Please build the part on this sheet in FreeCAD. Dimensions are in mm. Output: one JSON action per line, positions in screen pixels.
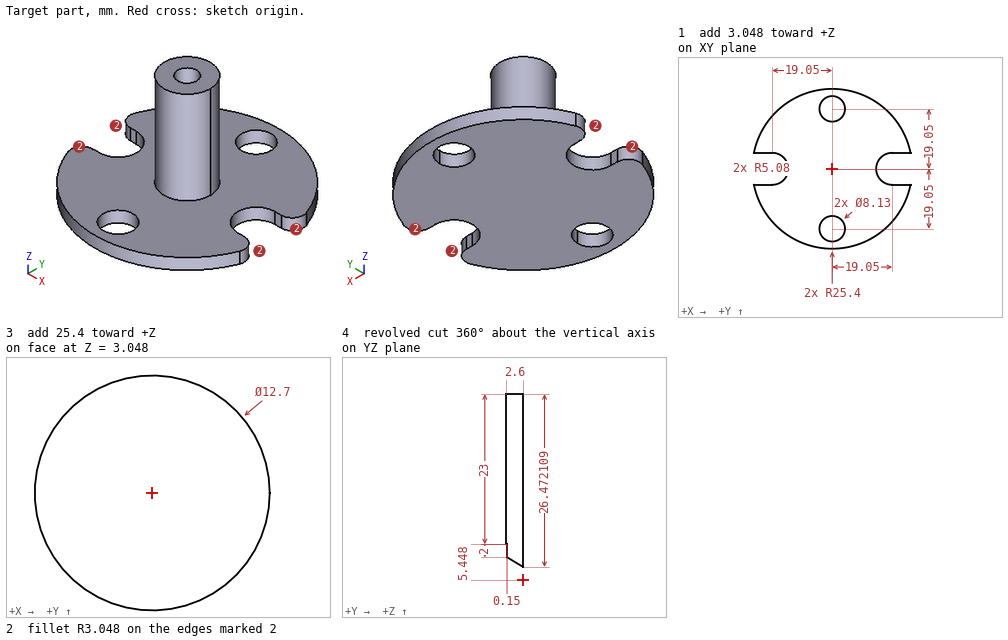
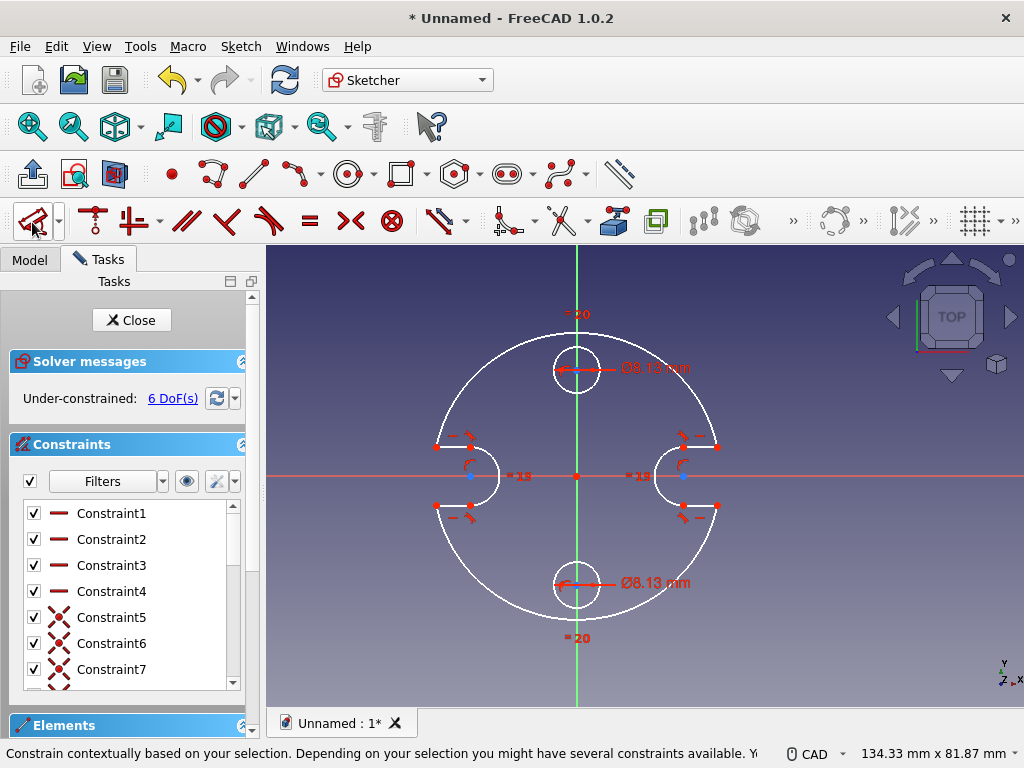
{"action": "scroll", "coordinate": [494, 494], "scroll_direction": "up", "scroll_amount": 2}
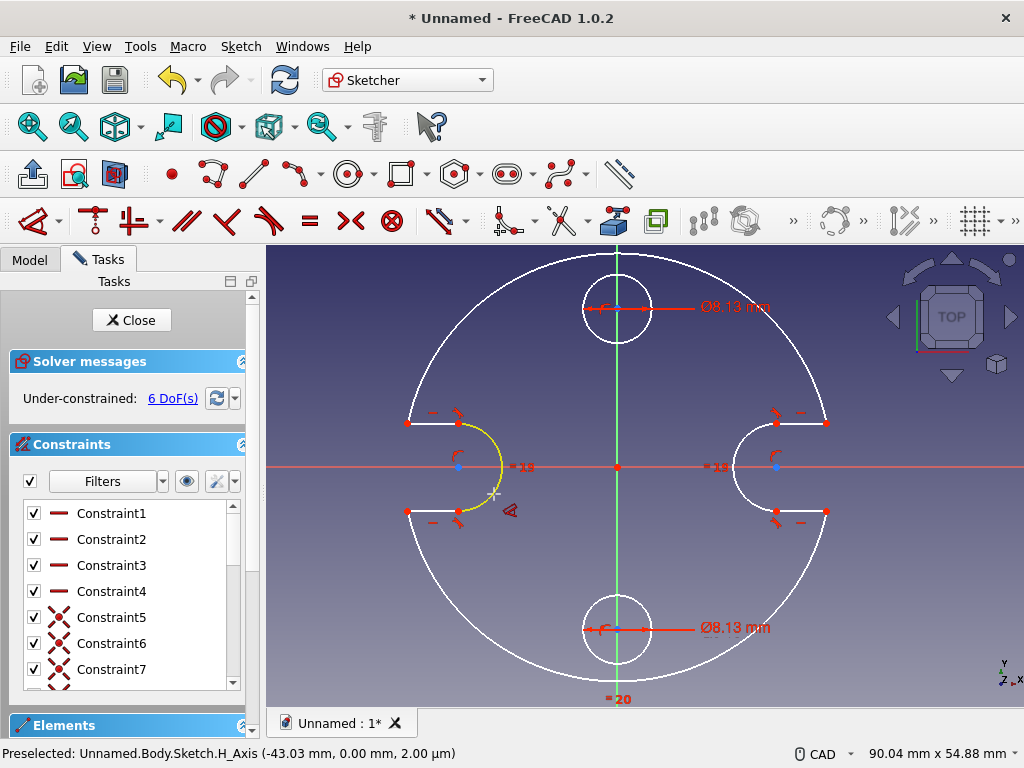
{"action": "left_click", "coordinate": [494, 493]}
{"action": "left_click", "coordinate": [520, 512]}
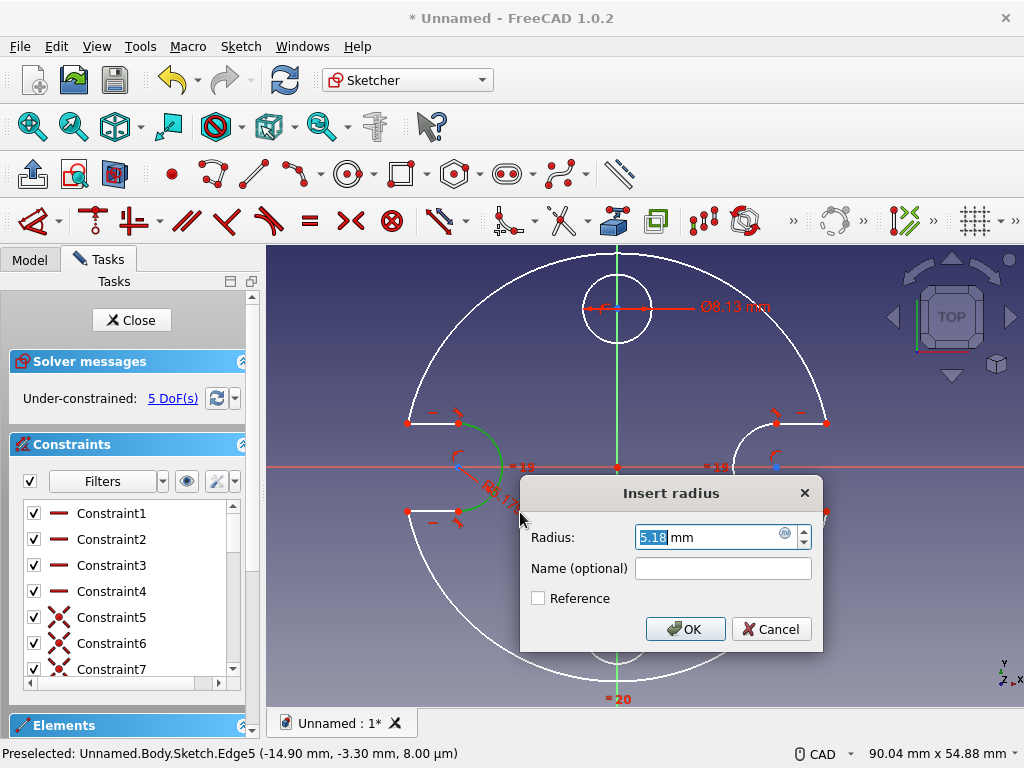
{"action": "type", "text": "5.08"}
{"action": "key", "text": "Return"}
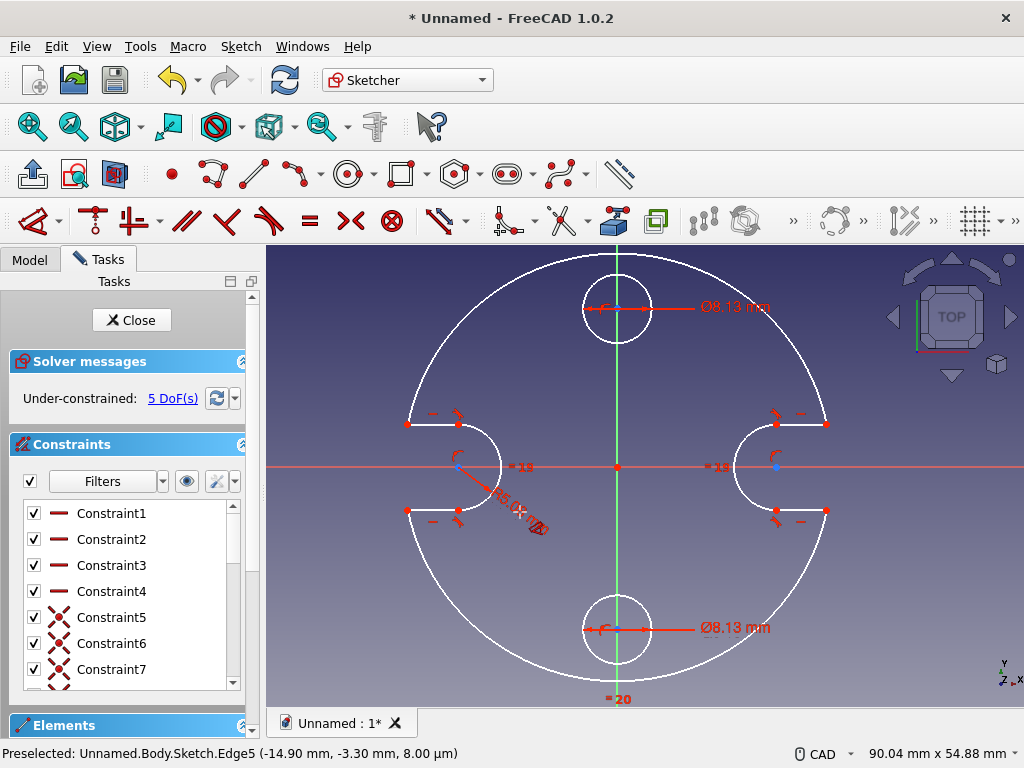
{"action": "left_click", "coordinate": [506, 650]}
{"action": "left_click", "coordinate": [489, 677]}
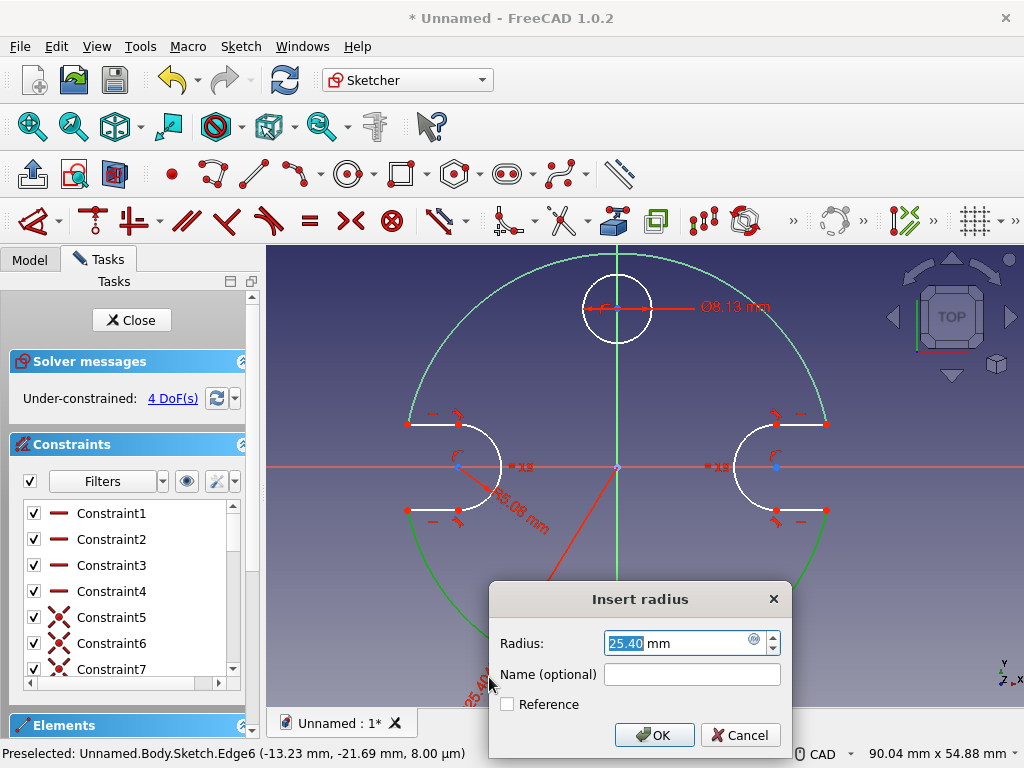
{"action": "type", "text": "25.4"}
{"action": "key", "text": "Return"}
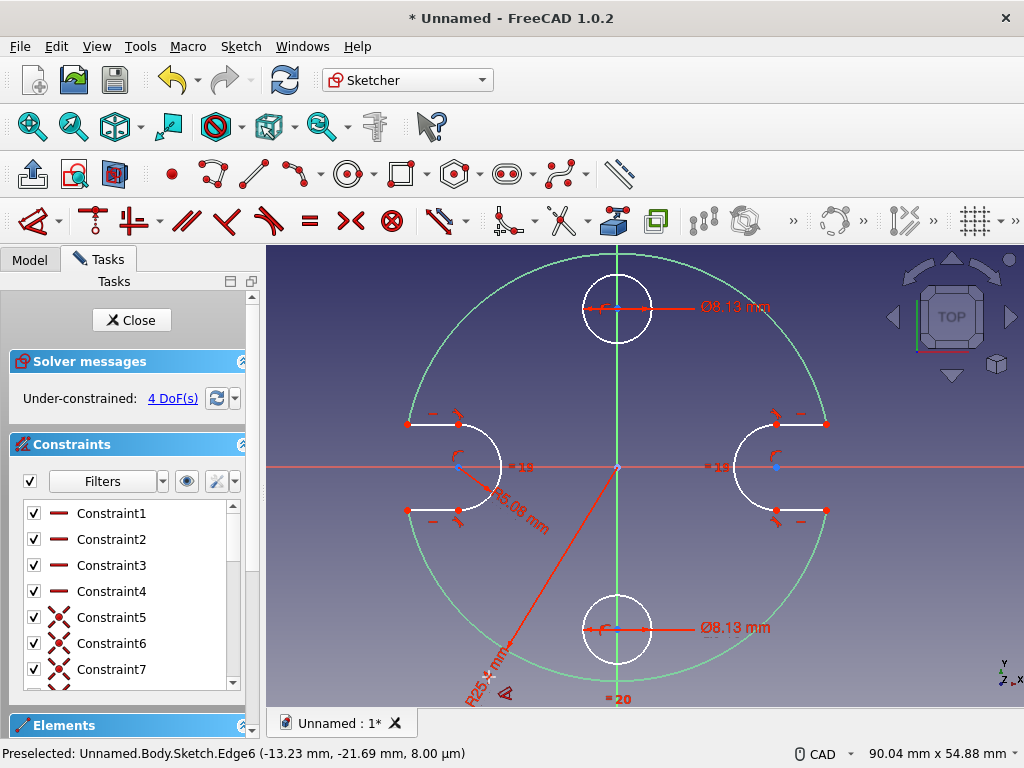
{"action": "left_click", "coordinate": [617, 630]}
{"action": "left_click", "coordinate": [651, 549]}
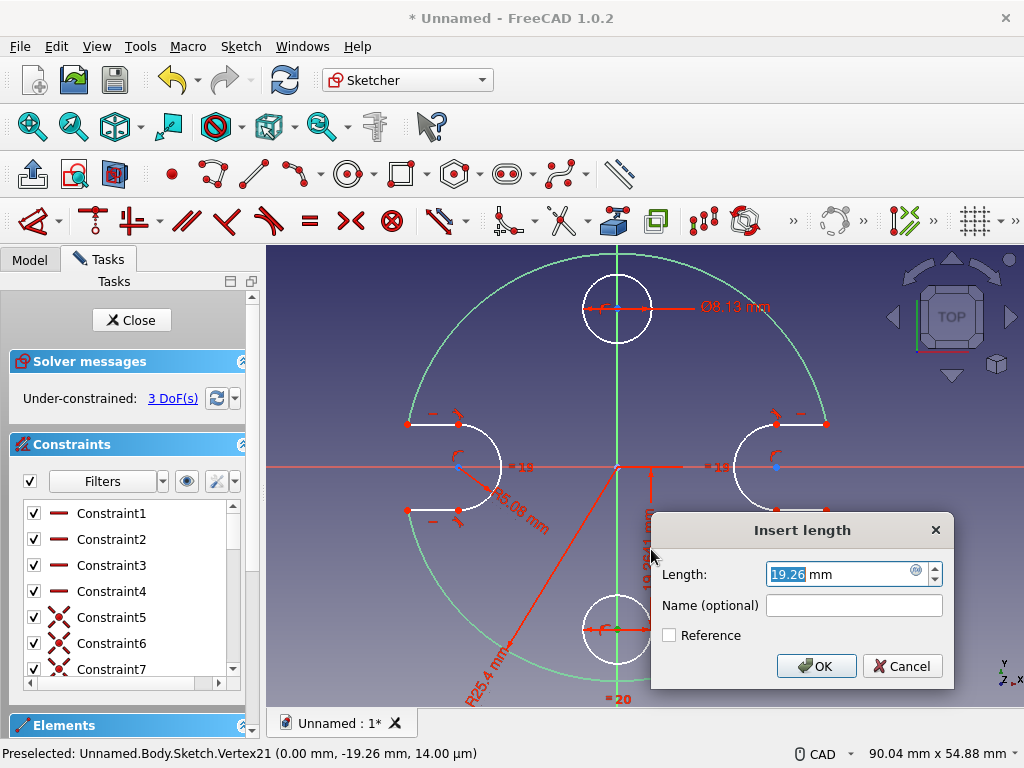
{"action": "type", "text": "19.05"}
{"action": "key", "text": "Return"}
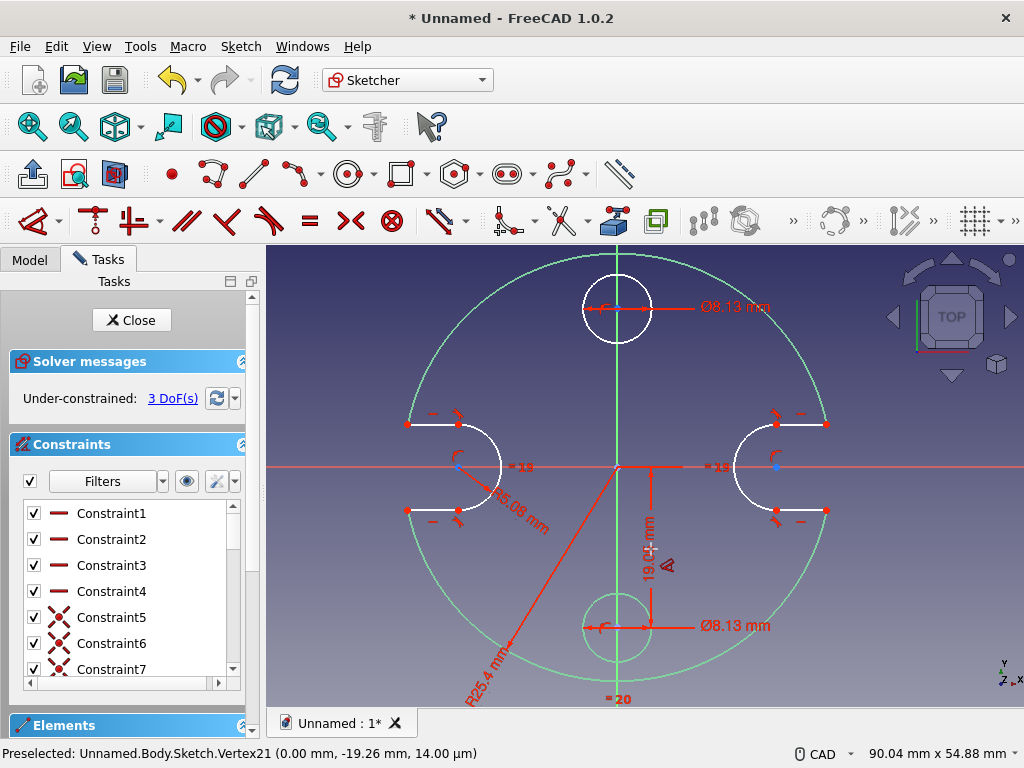
{"action": "left_click", "coordinate": [617, 309]}
{"action": "left_click", "coordinate": [651, 388]}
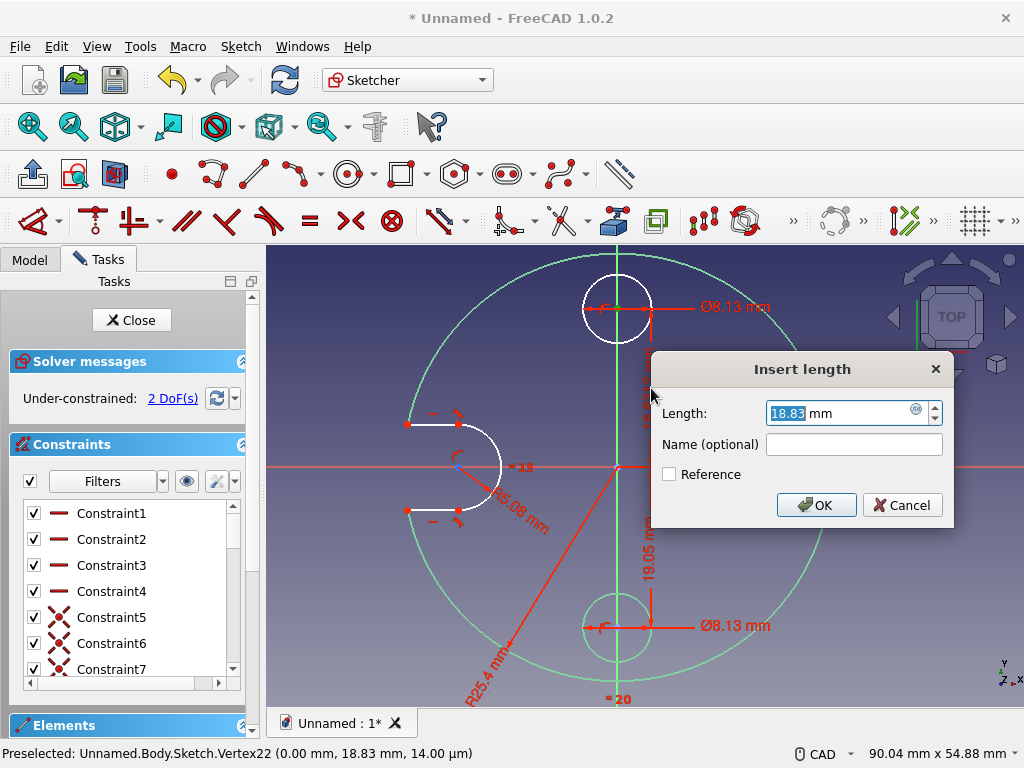
{"action": "type", "text": "19.05"}
{"action": "key", "text": "Return"}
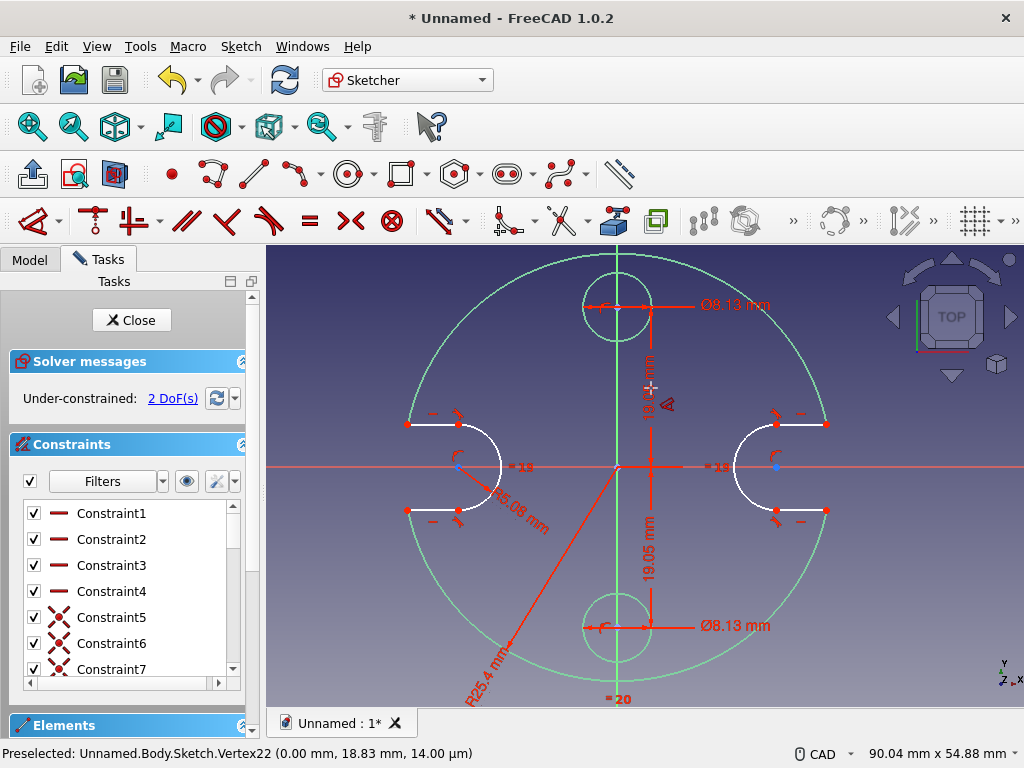
{"action": "left_click", "coordinate": [458, 425]}
{"action": "left_click", "coordinate": [538, 391]}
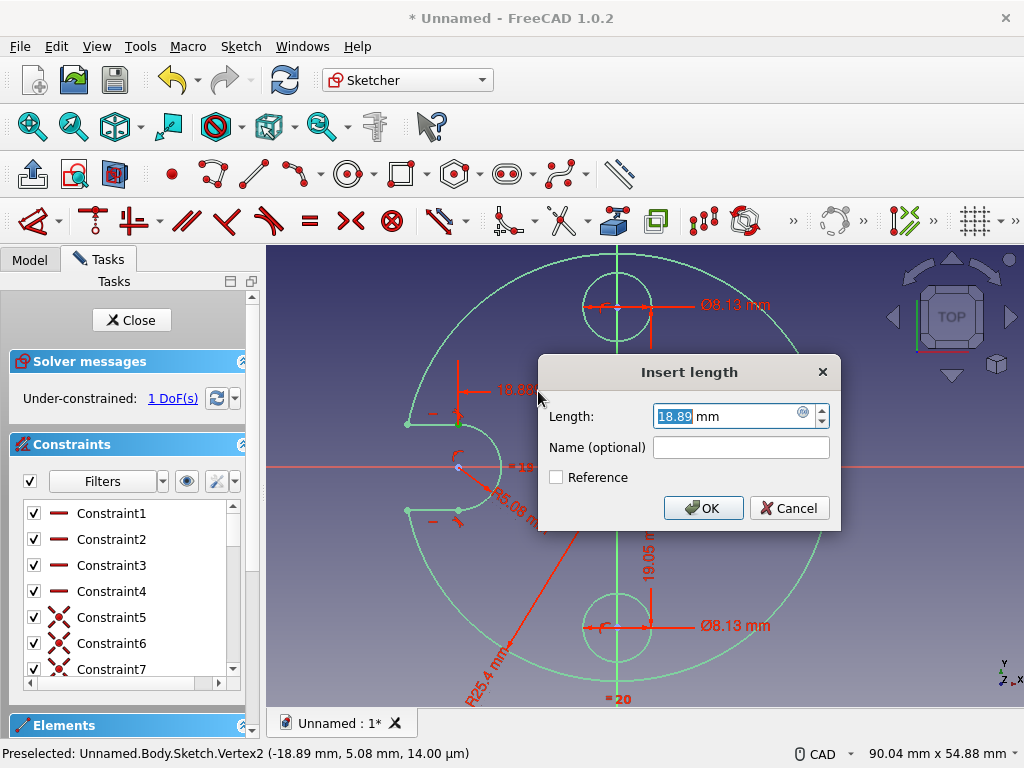
{"action": "type", "text": "19.05"}
{"action": "key", "text": "Return"}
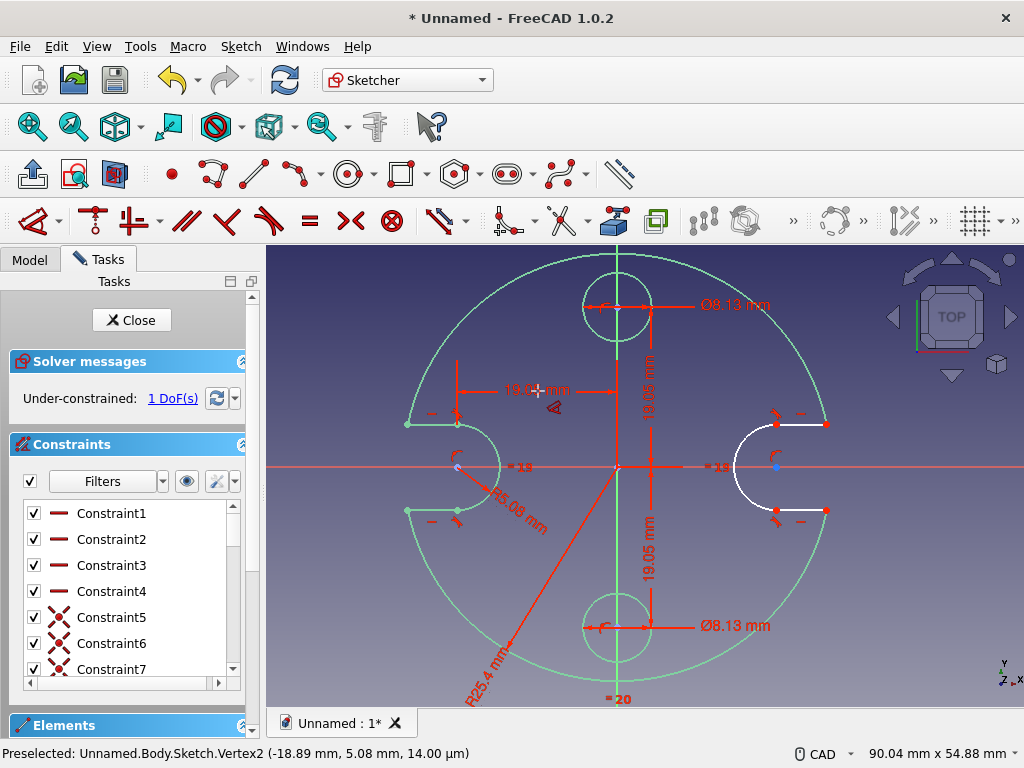
{"action": "left_click", "coordinate": [777, 510]}
{"action": "left_click", "coordinate": [734, 544]}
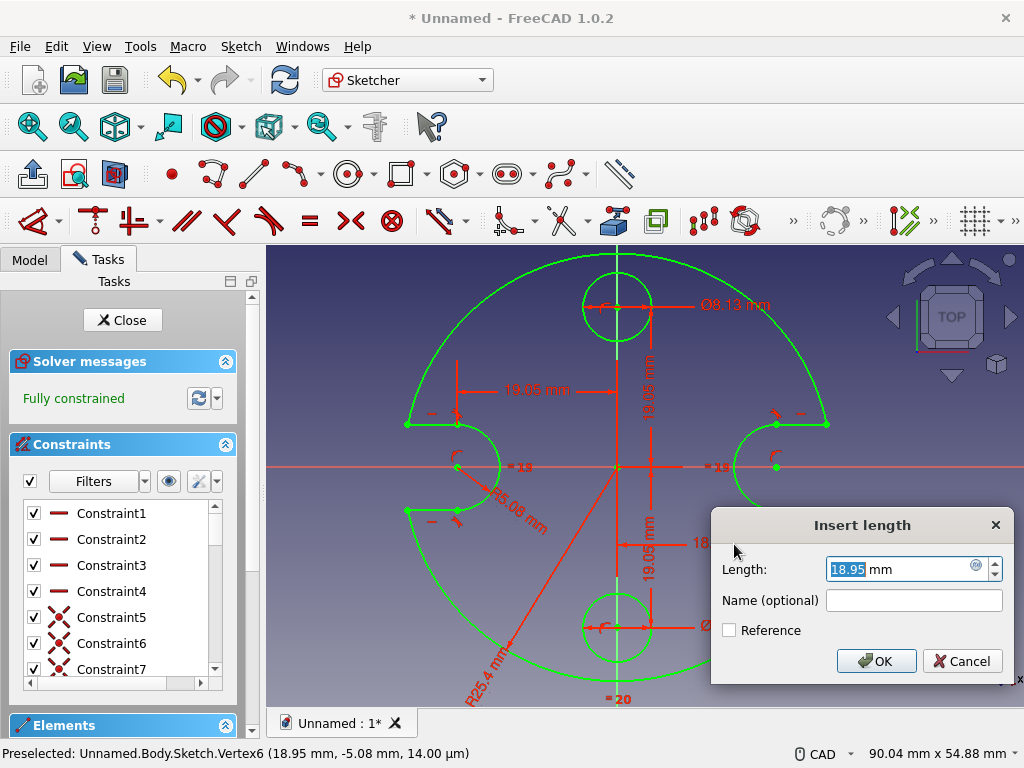
{"action": "type", "text": "19.05"}
{"action": "key", "text": "Return"}
{"action": "key", "text": "Escape"}